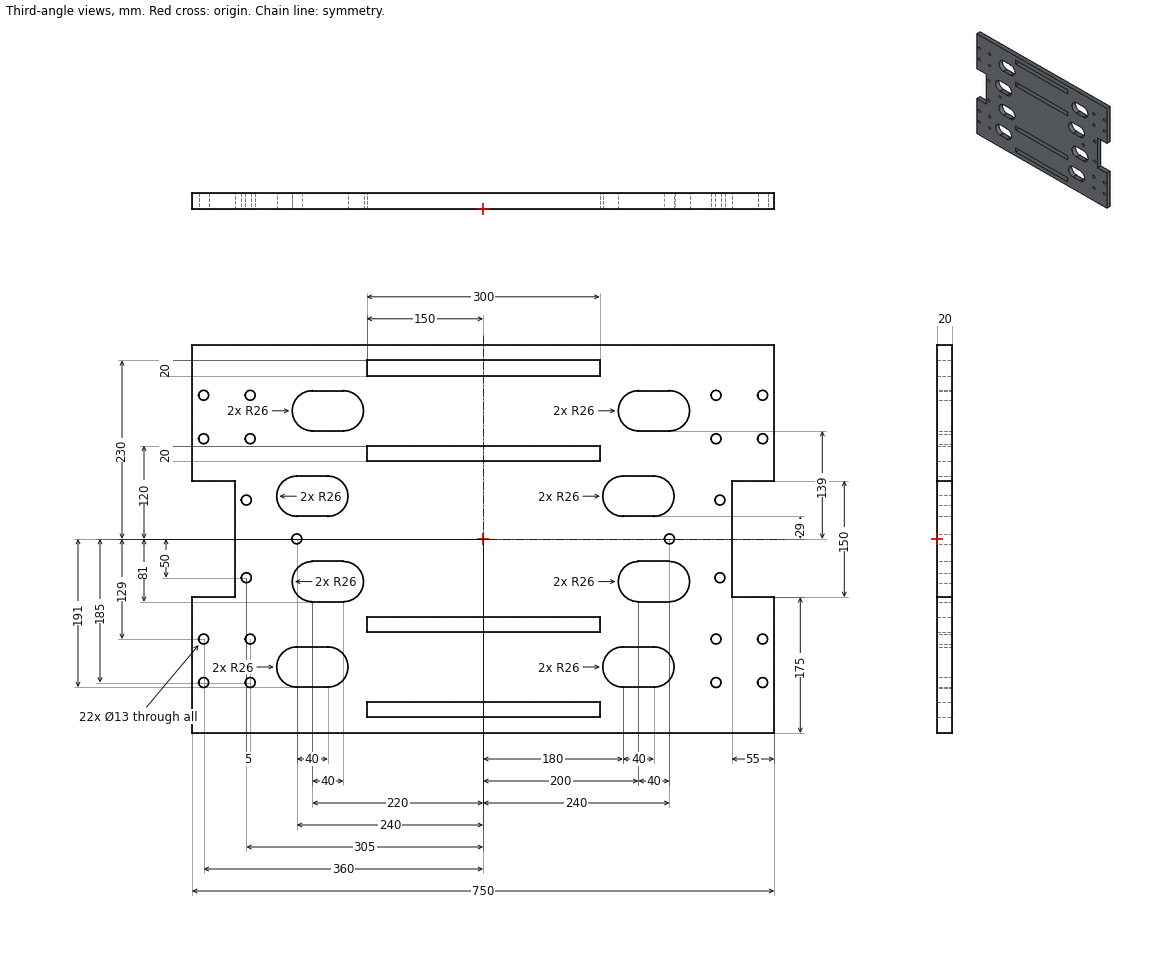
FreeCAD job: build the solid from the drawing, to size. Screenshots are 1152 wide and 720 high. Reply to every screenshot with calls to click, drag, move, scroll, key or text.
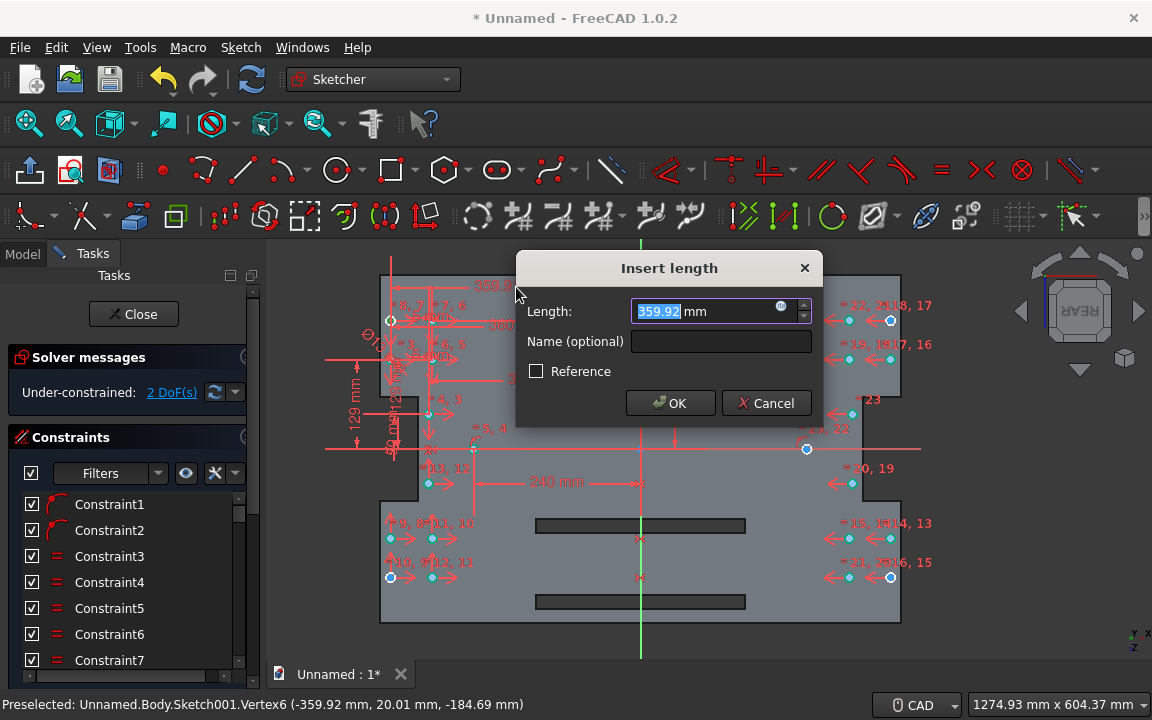
text(360)
key(Return)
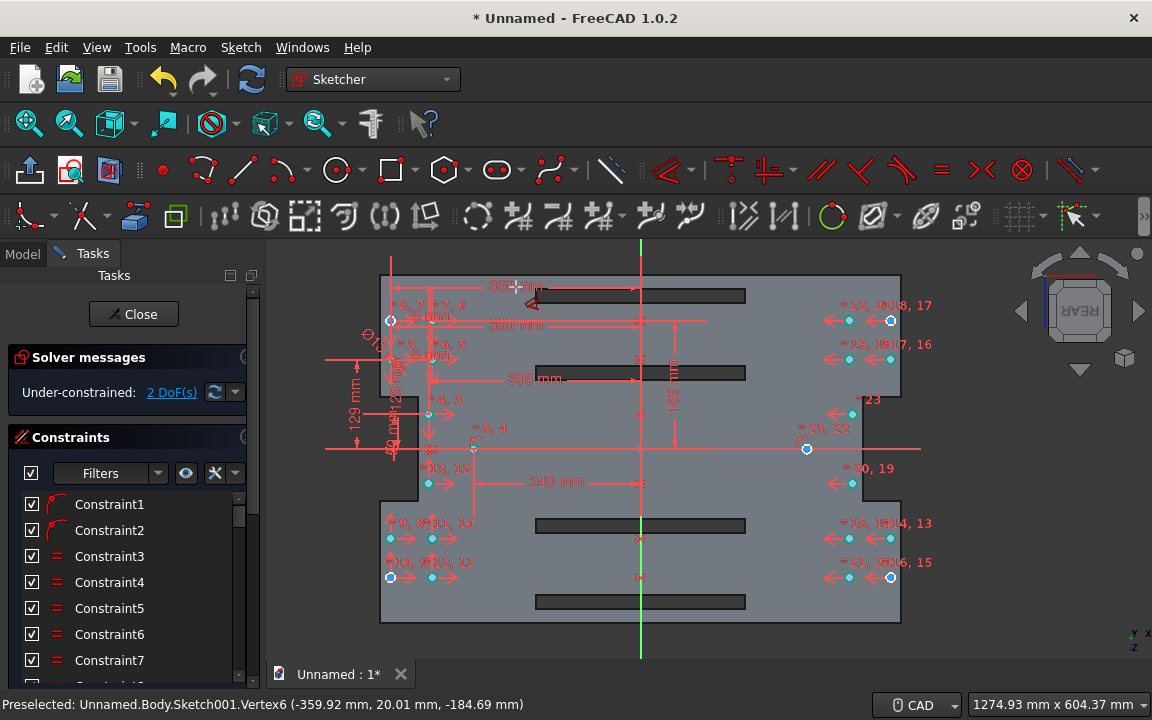
click(391, 321)
click(675, 356)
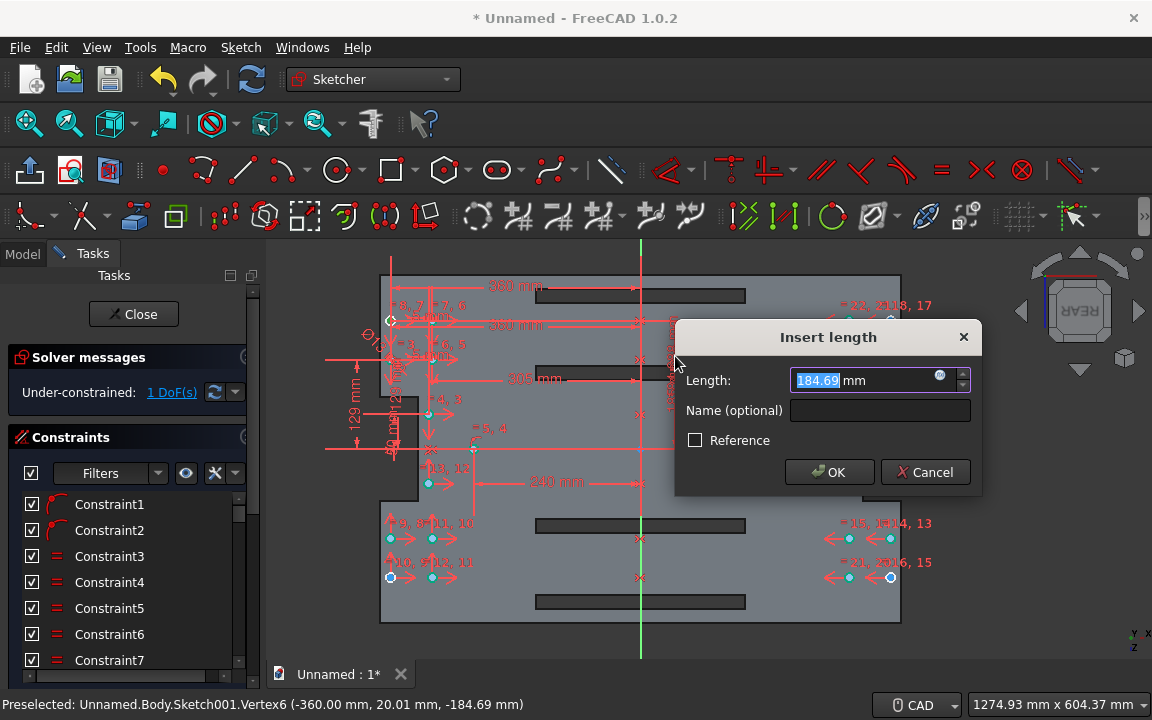
text(185)
key(Return)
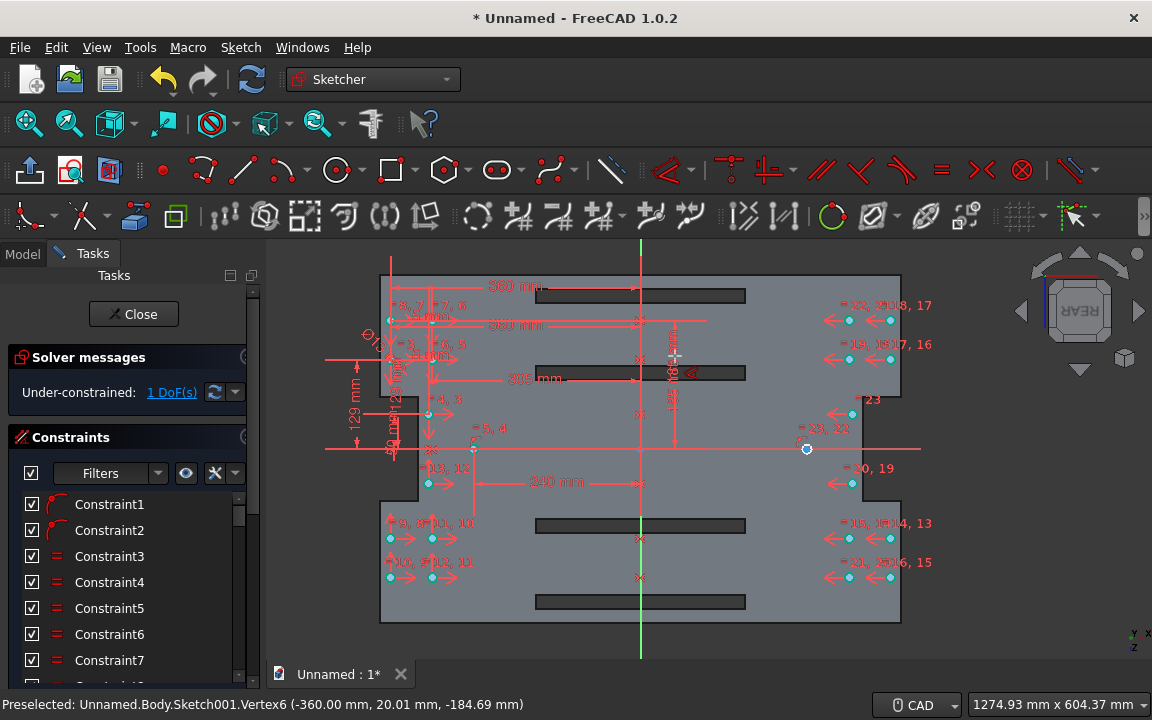
click(807, 449)
click(724, 483)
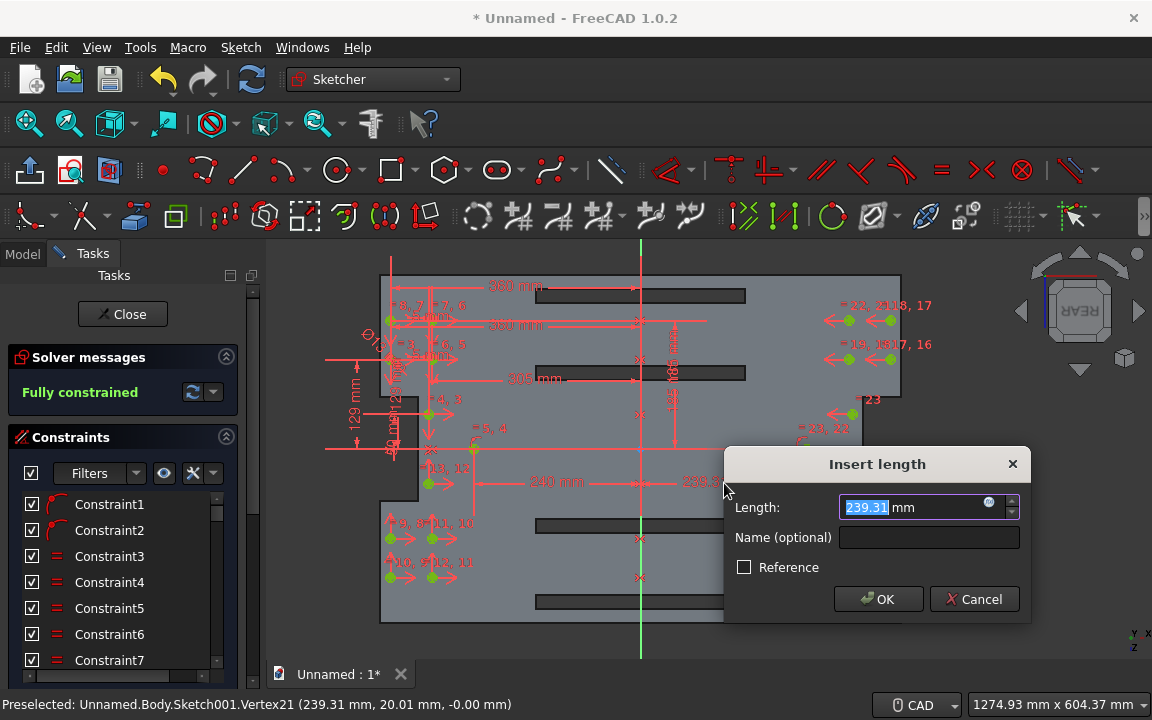
text(240)
key(Return)
key(Escape)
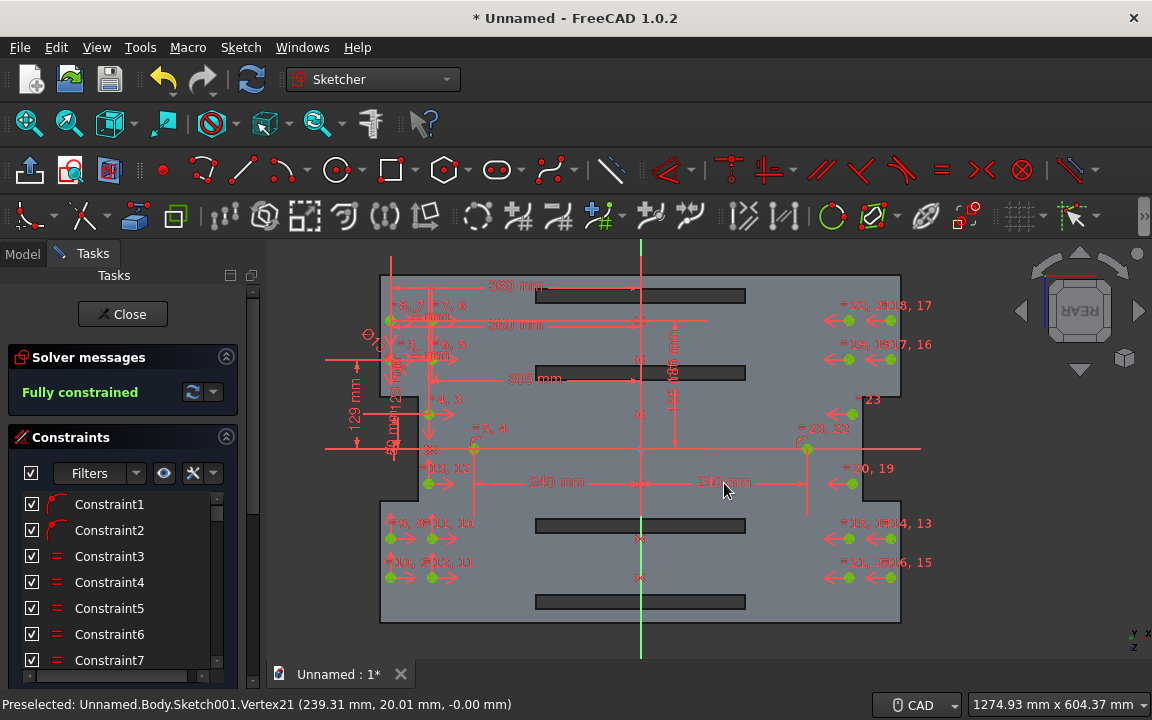
click(123, 314)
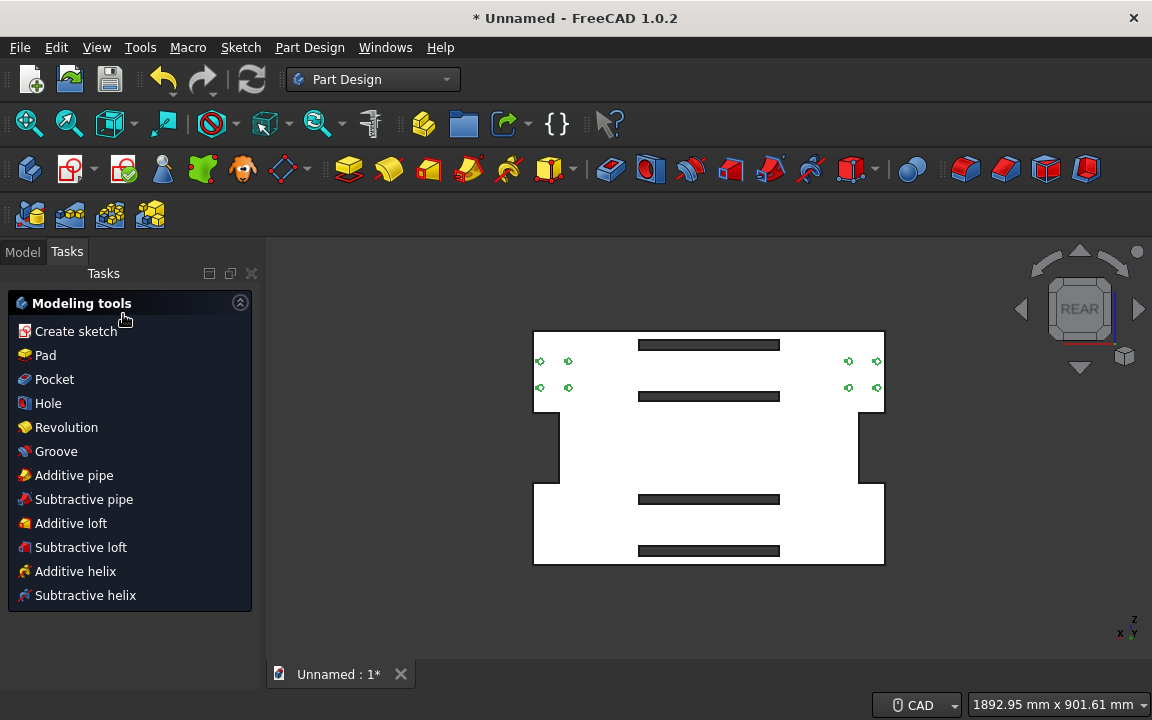
click(652, 170)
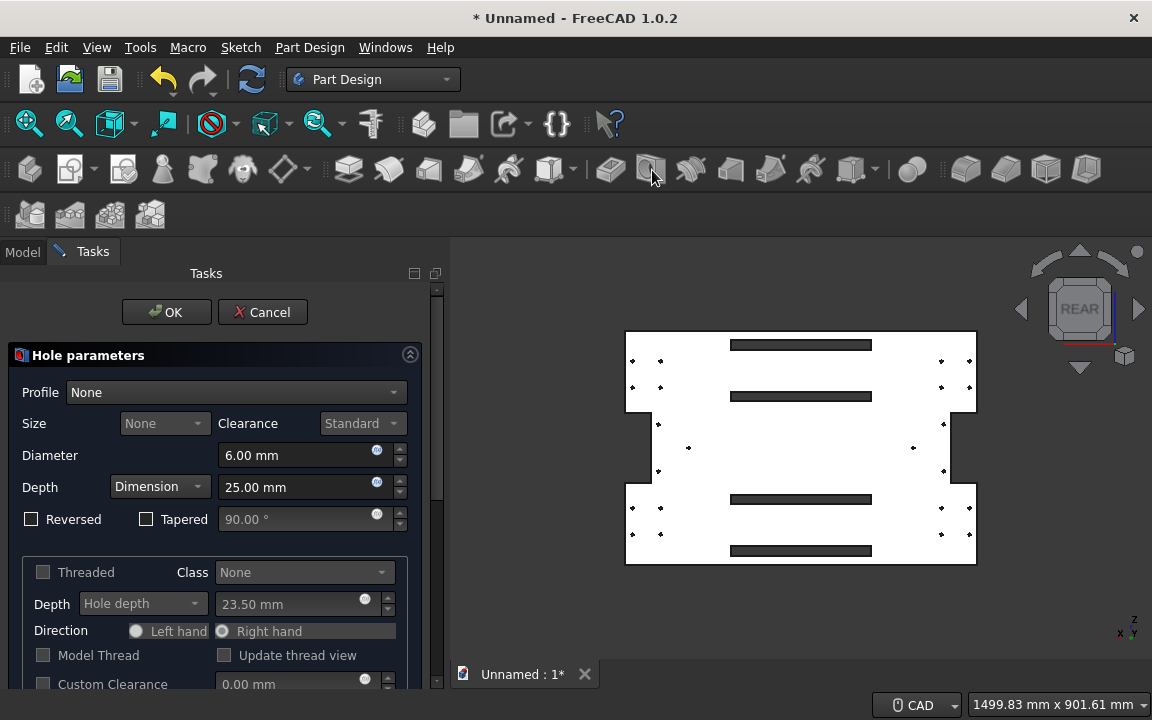
triple_click(305, 455)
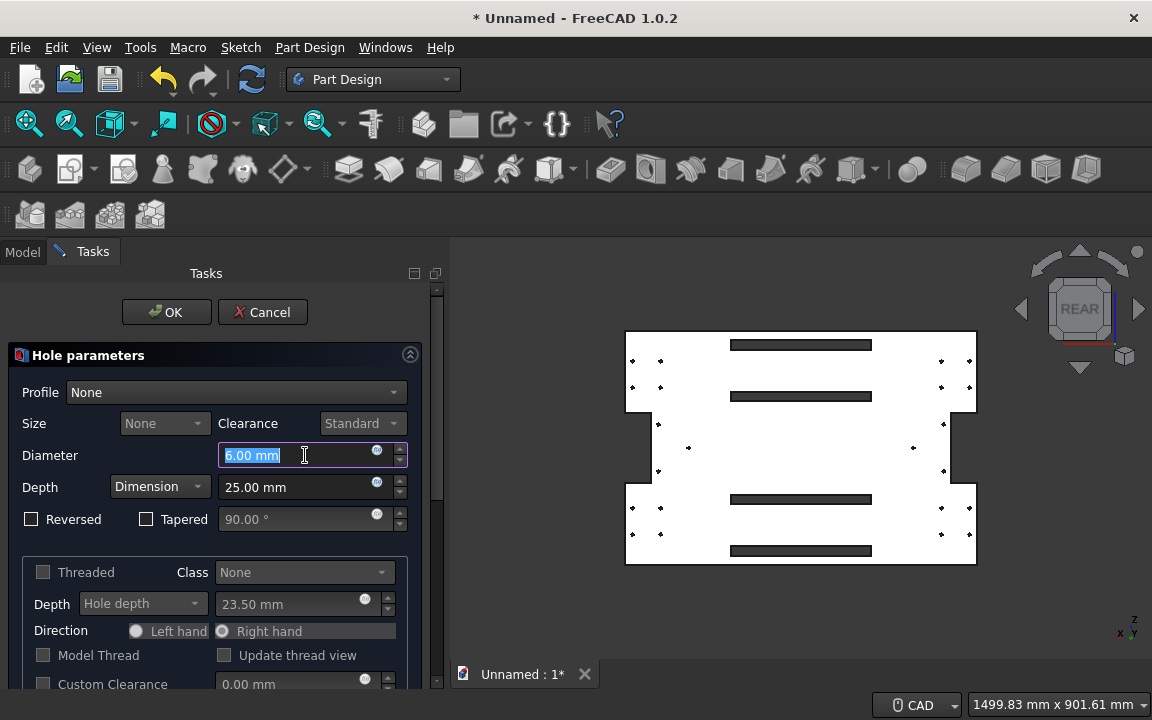
text(13)
key(Tab)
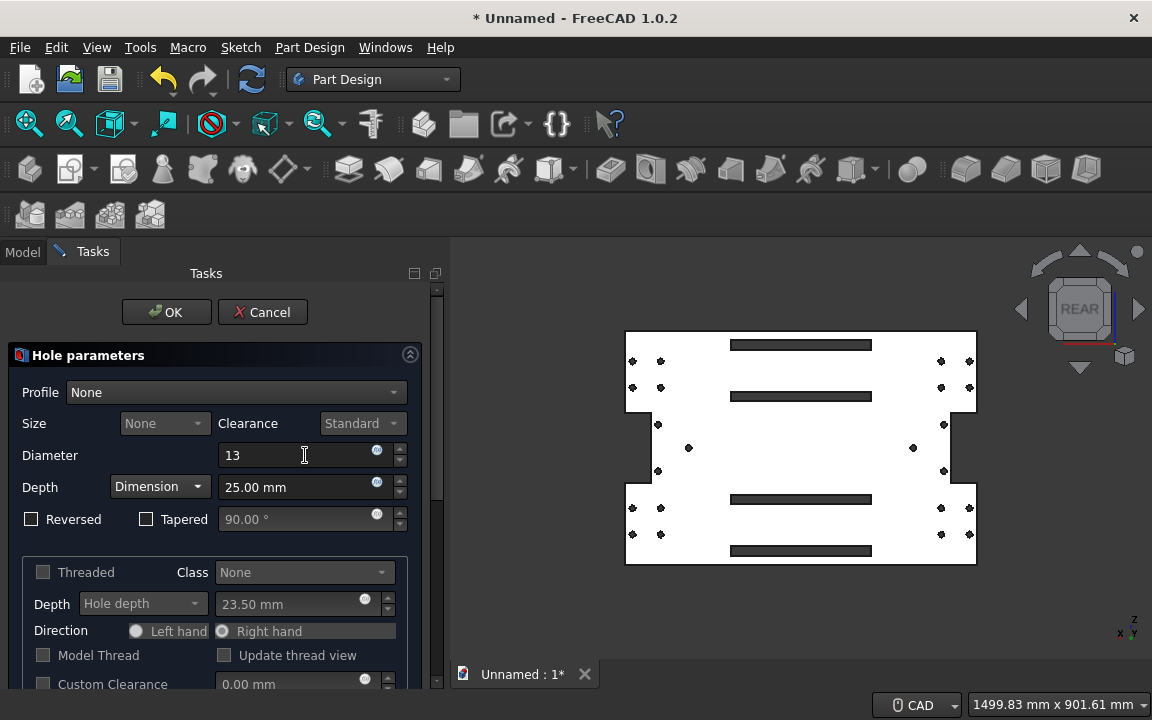
click(161, 486)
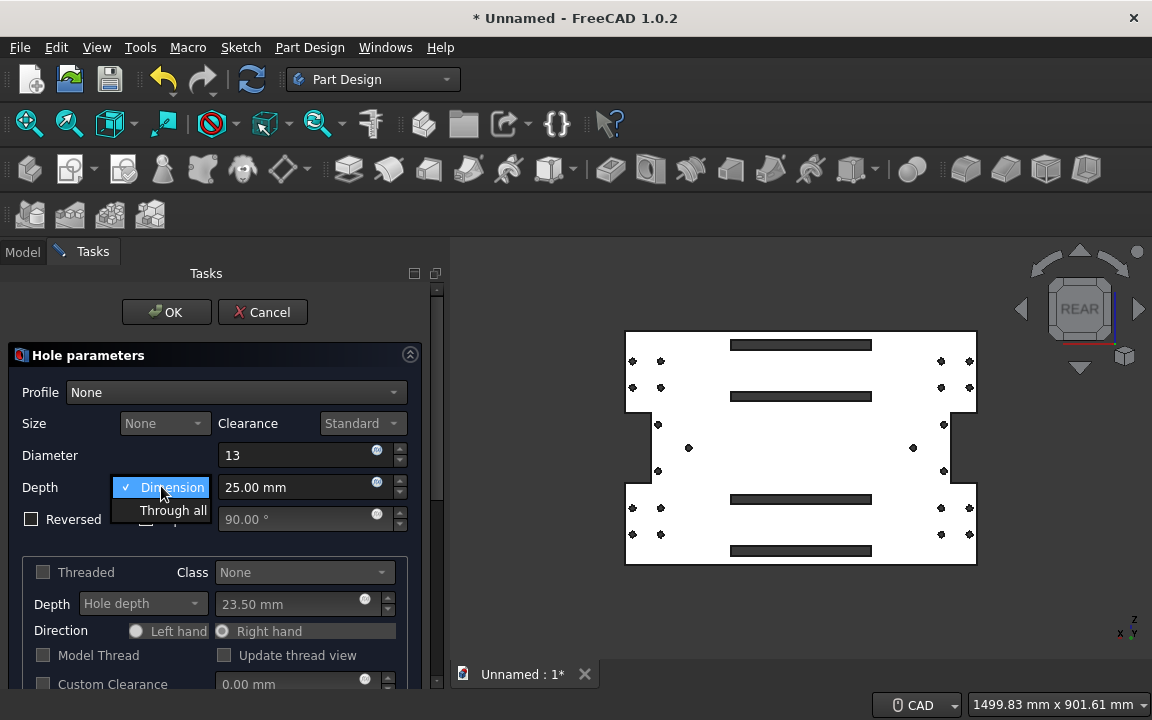
click(160, 510)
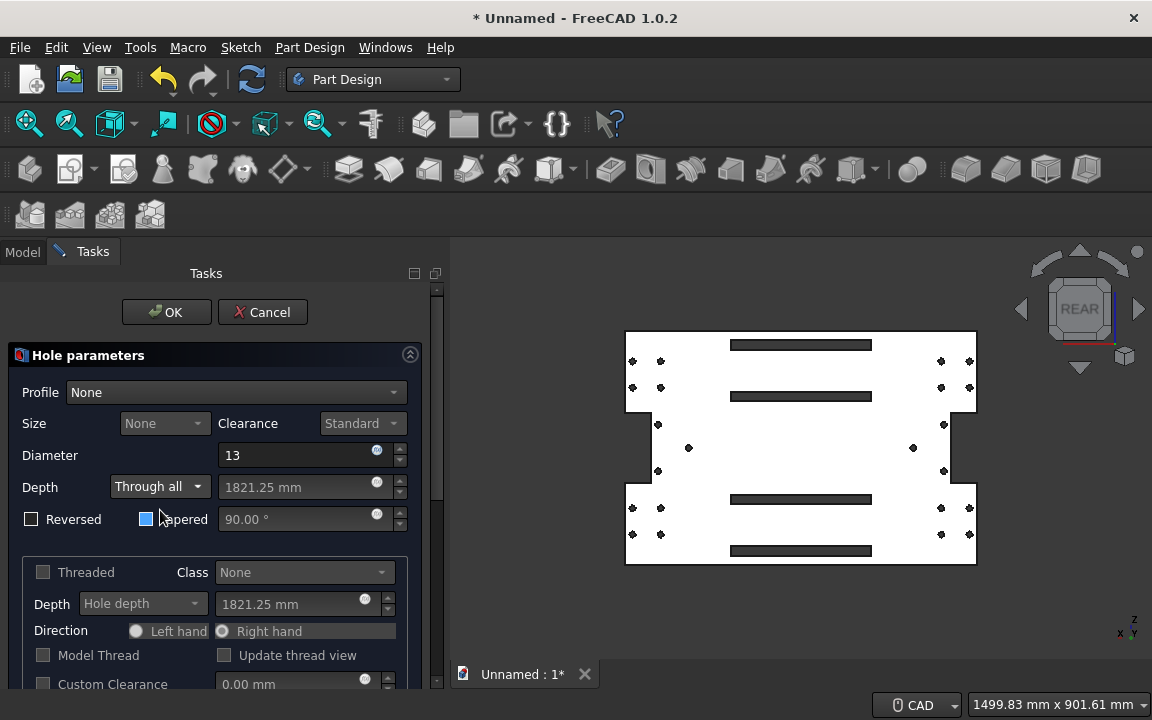
click(167, 312)